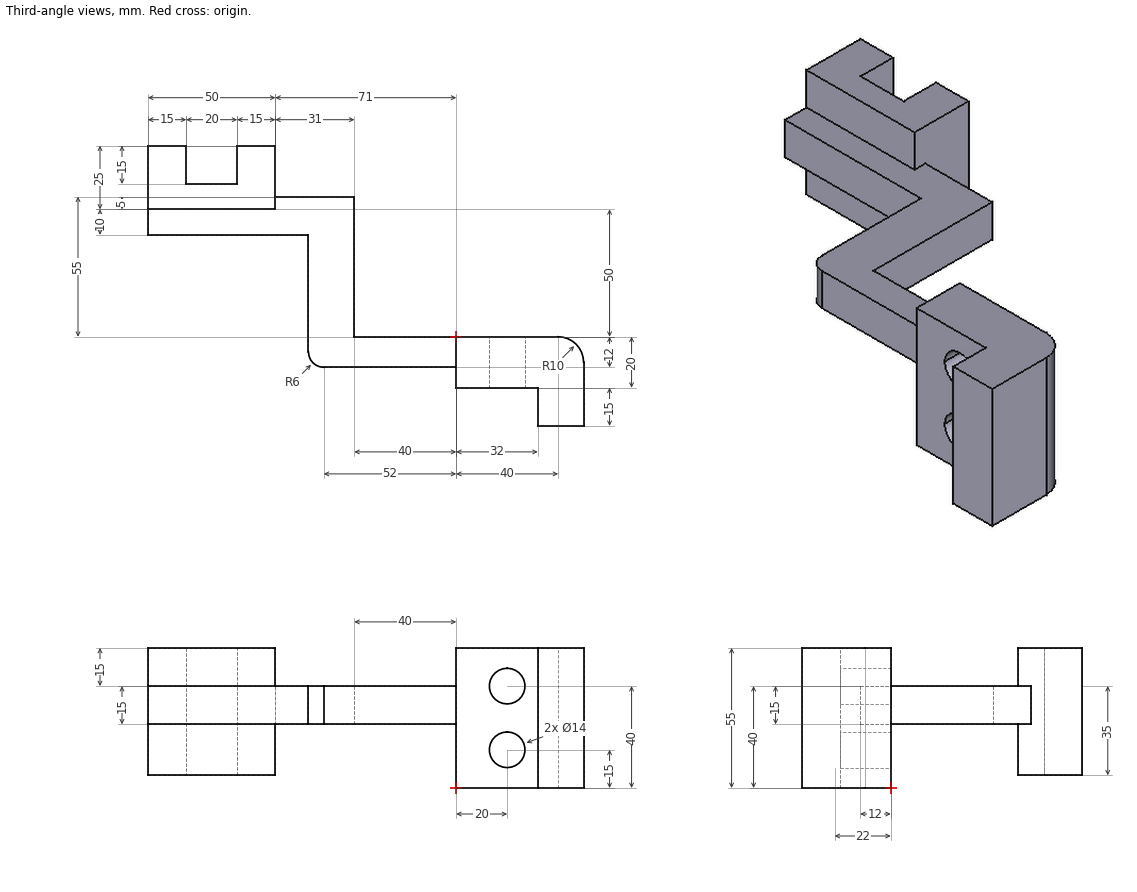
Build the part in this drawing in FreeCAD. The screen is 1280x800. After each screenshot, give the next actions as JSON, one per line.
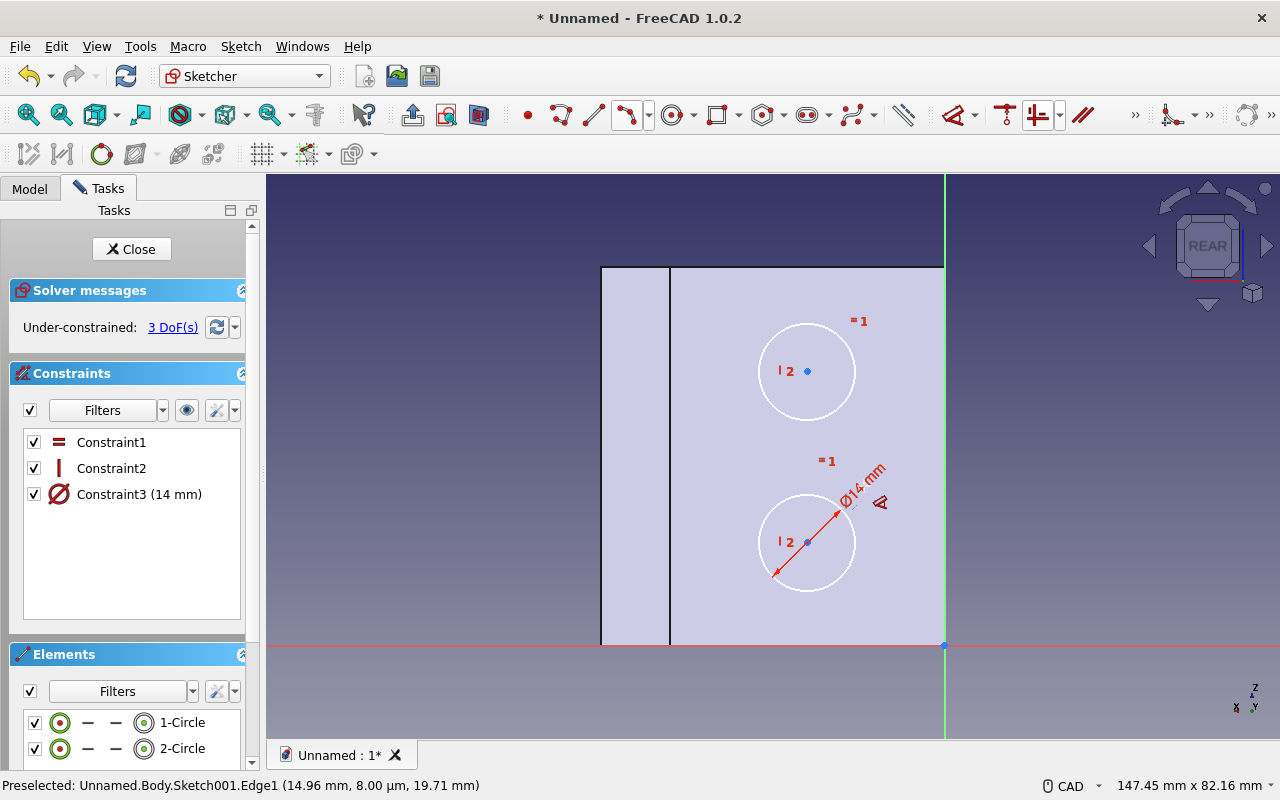
{"action": "left_click", "coordinate": [807, 543]}
{"action": "left_click", "coordinate": [876, 680]}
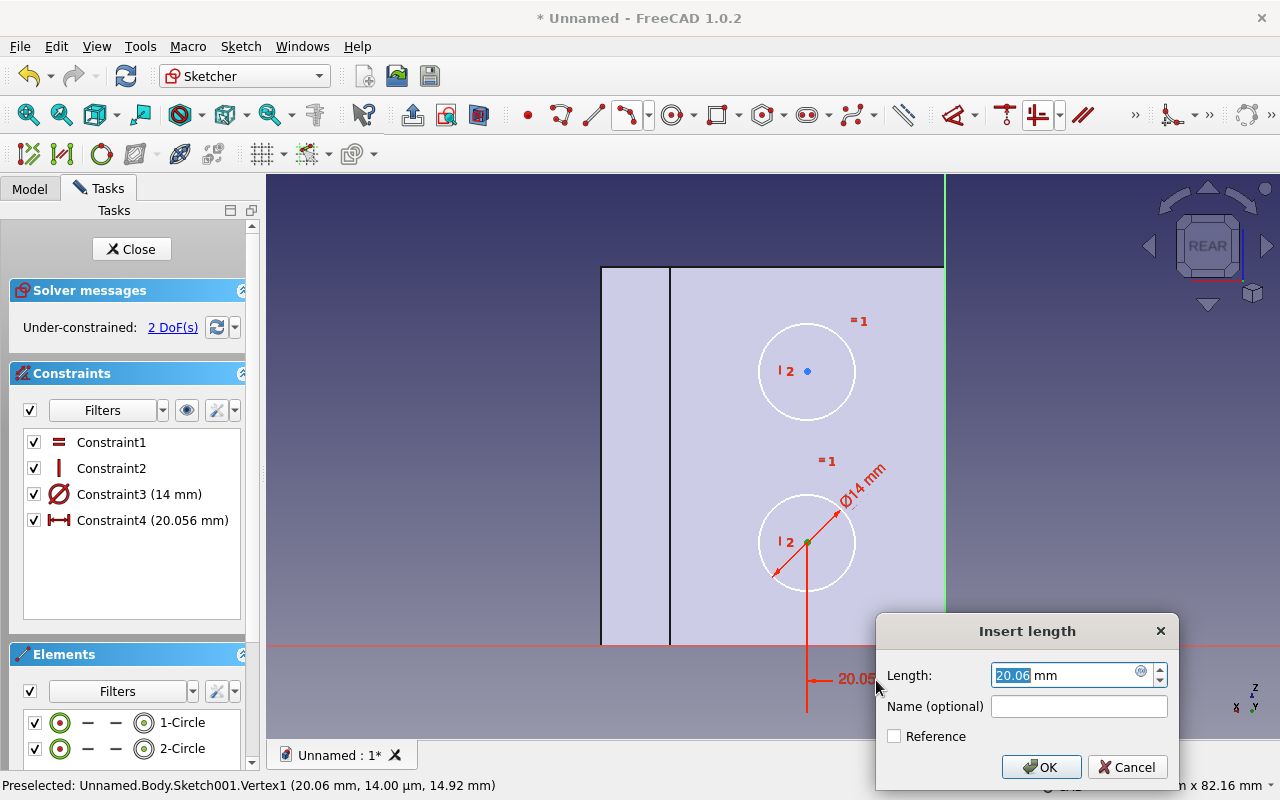
{"action": "type", "text": "20"}
{"action": "key", "text": "Return"}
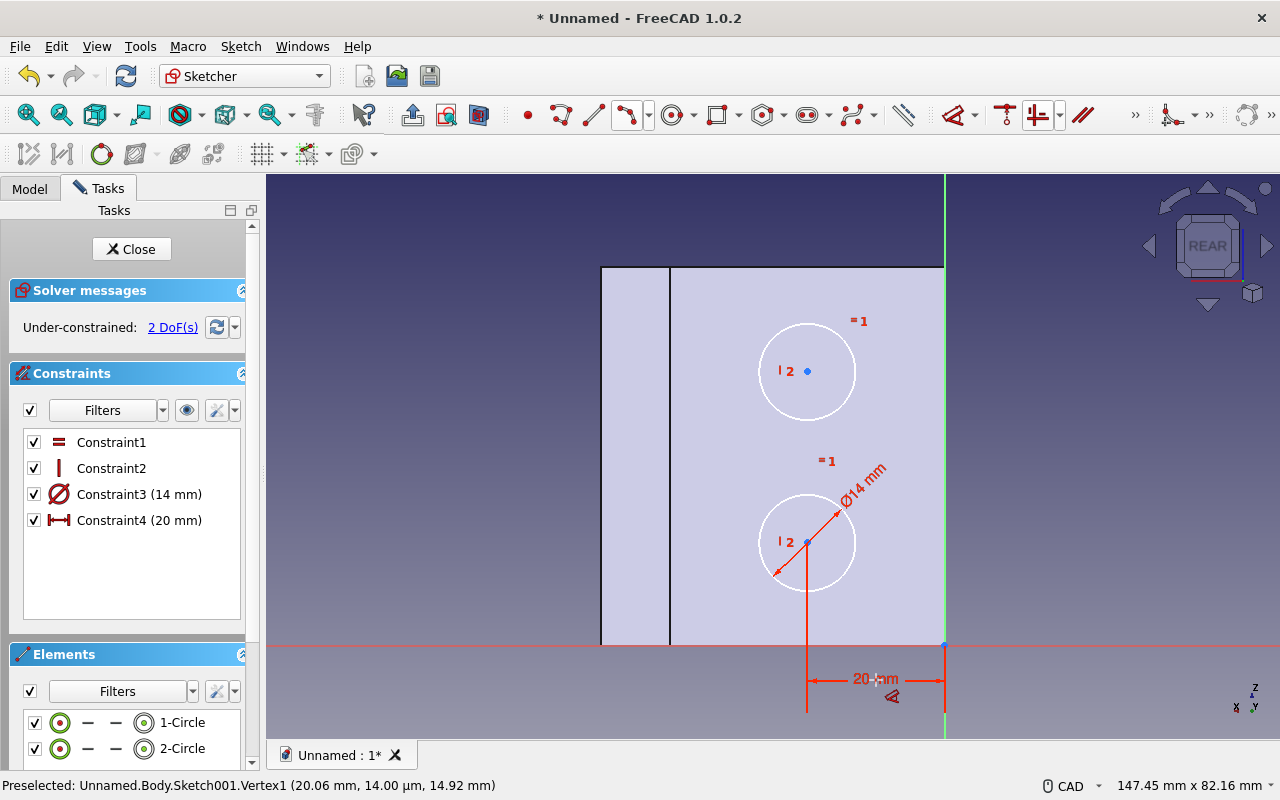
{"action": "left_click", "coordinate": [807, 543]}
{"action": "left_click", "coordinate": [979, 594]}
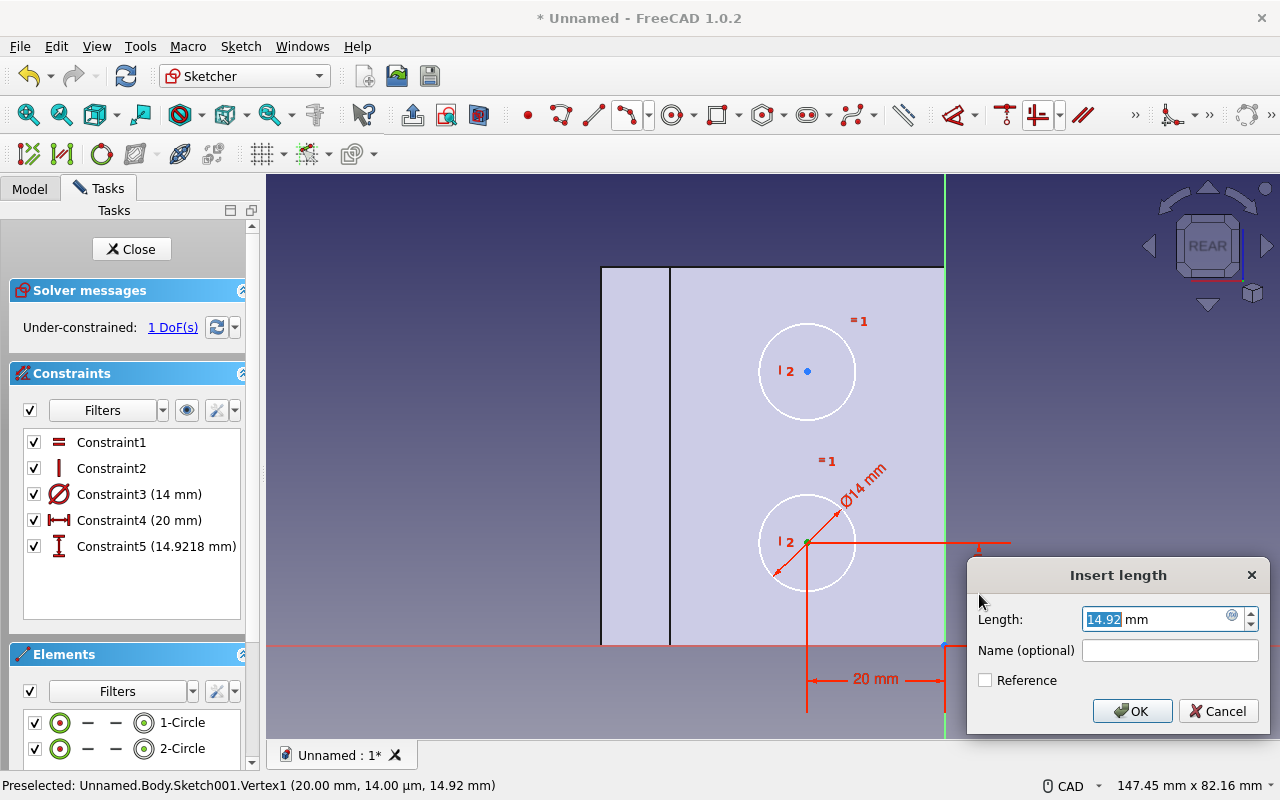
{"action": "type", "text": "15"}
{"action": "key", "text": "Return"}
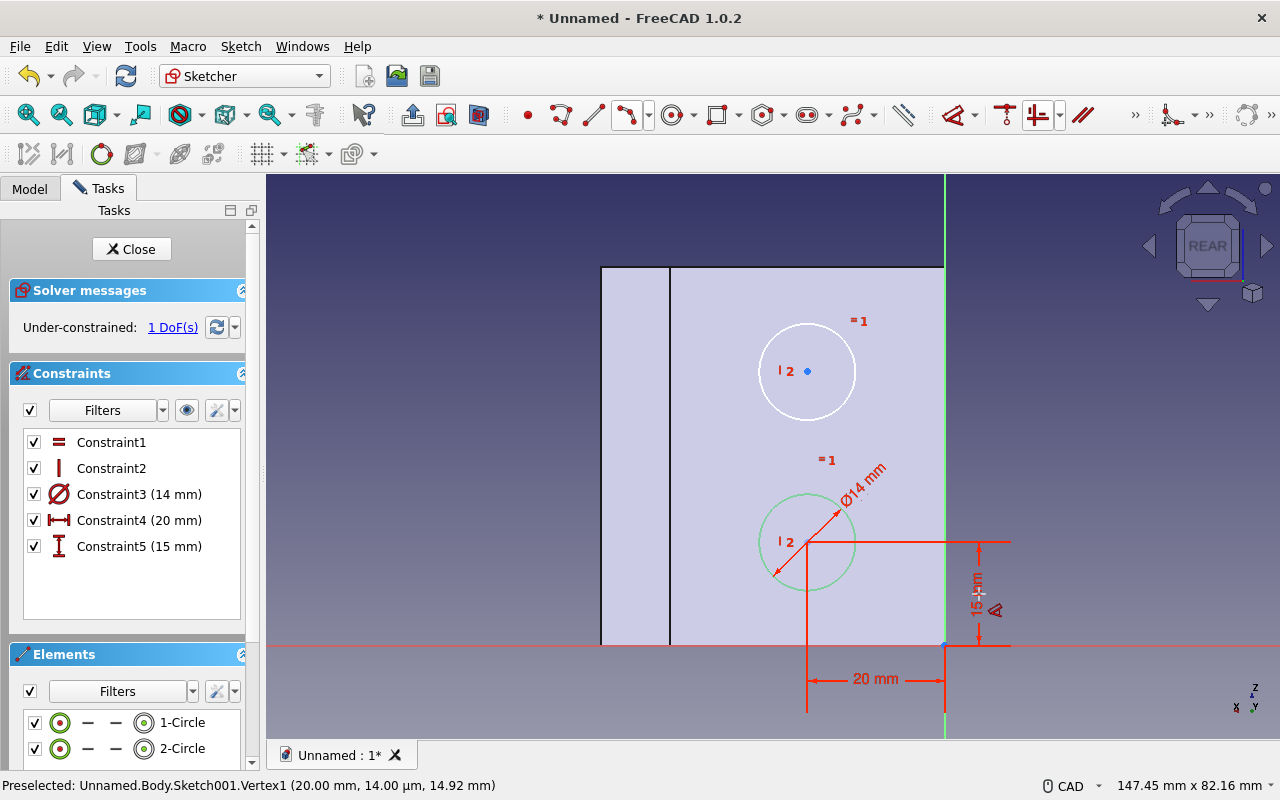
{"action": "left_click", "coordinate": [807, 372]}
{"action": "left_click", "coordinate": [979, 509]}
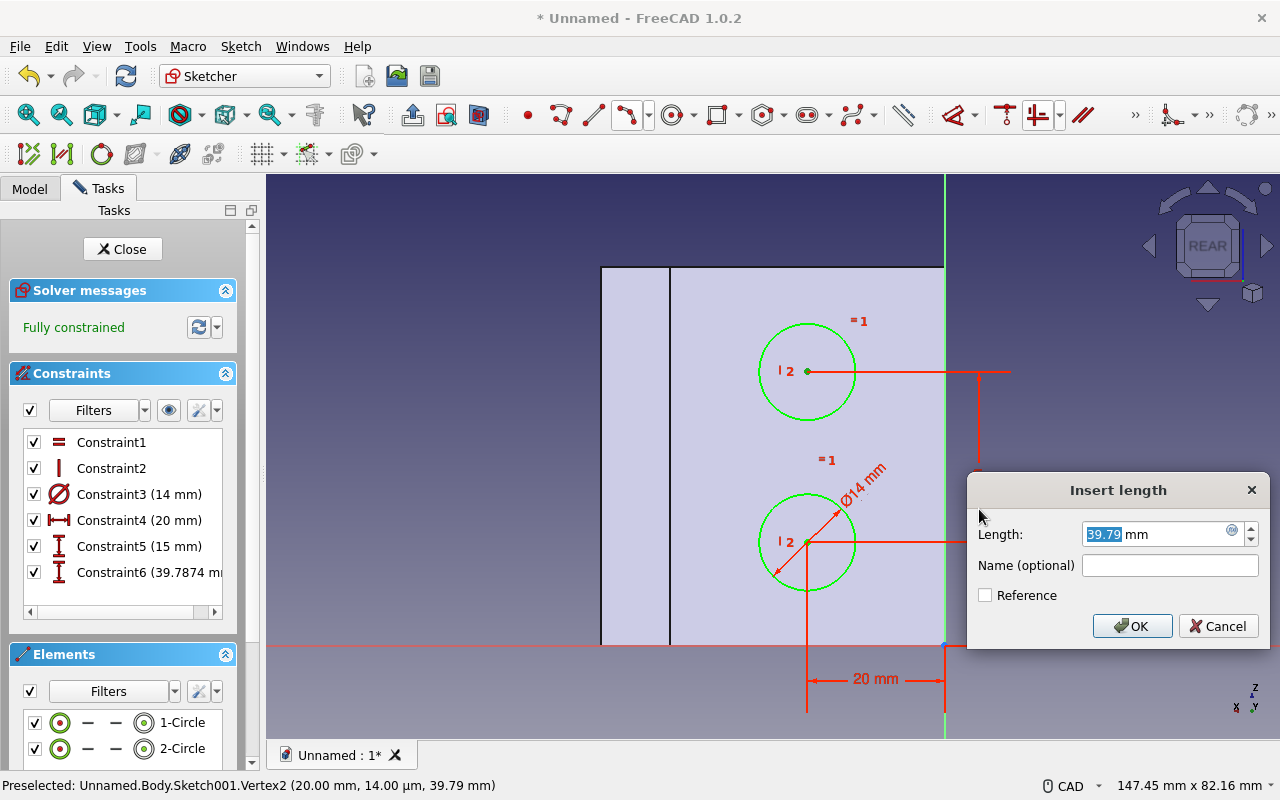
{"action": "type", "text": "40"}
{"action": "key", "text": "Return"}
{"action": "key", "text": "Escape"}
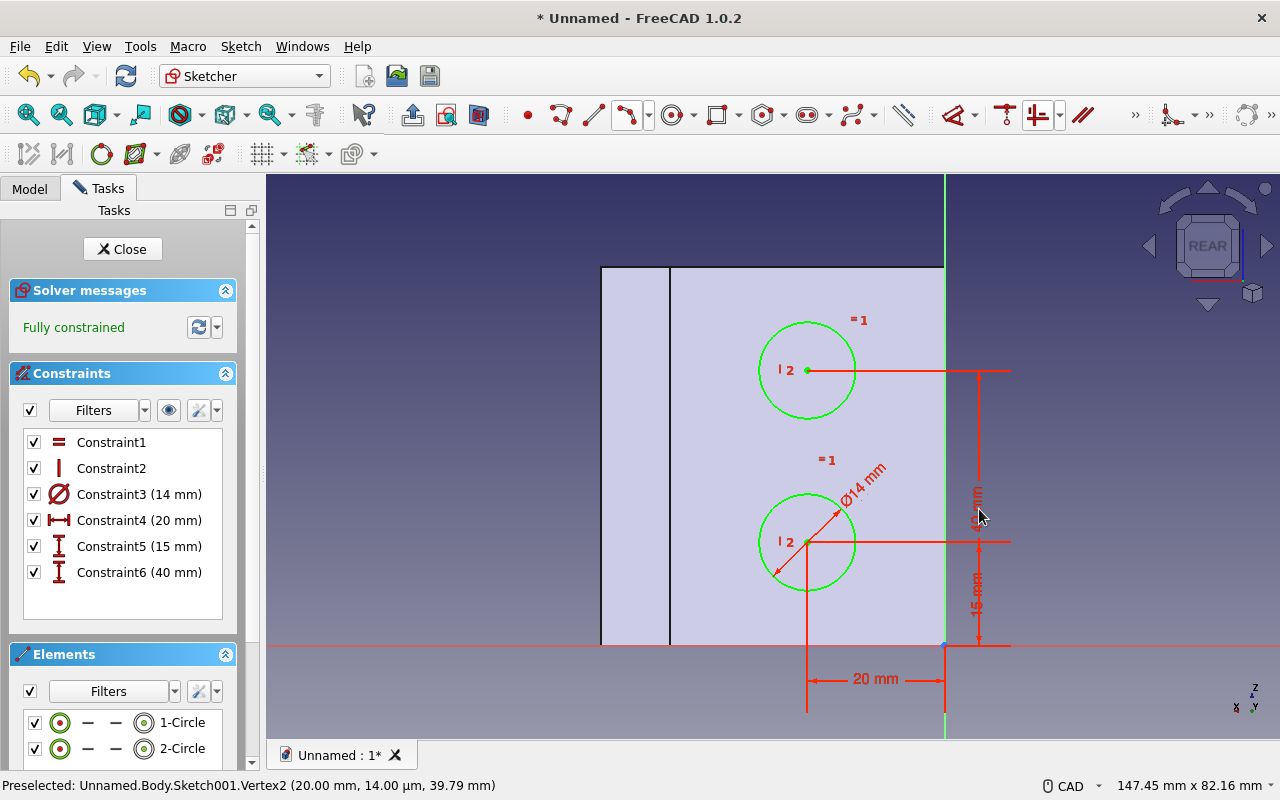
{"action": "left_click", "coordinate": [123, 249]}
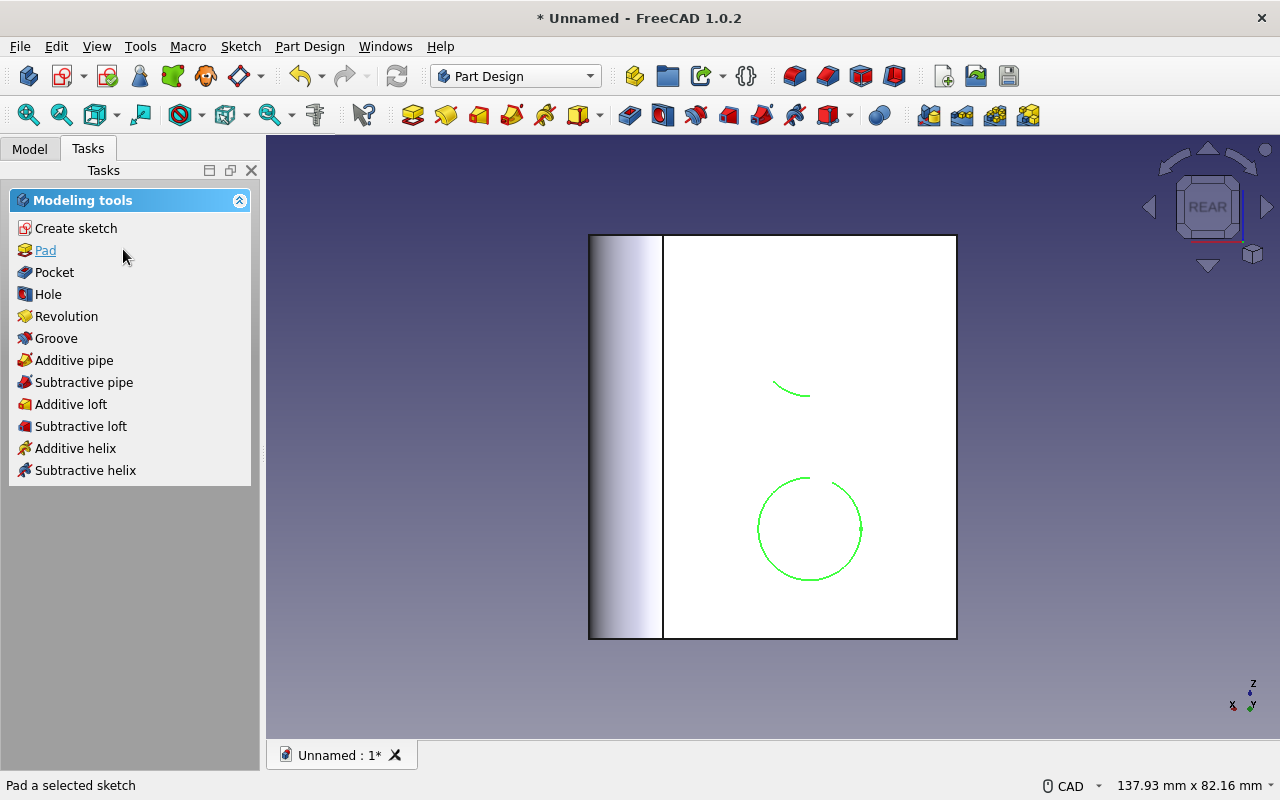
{"action": "left_click", "coordinate": [630, 116]}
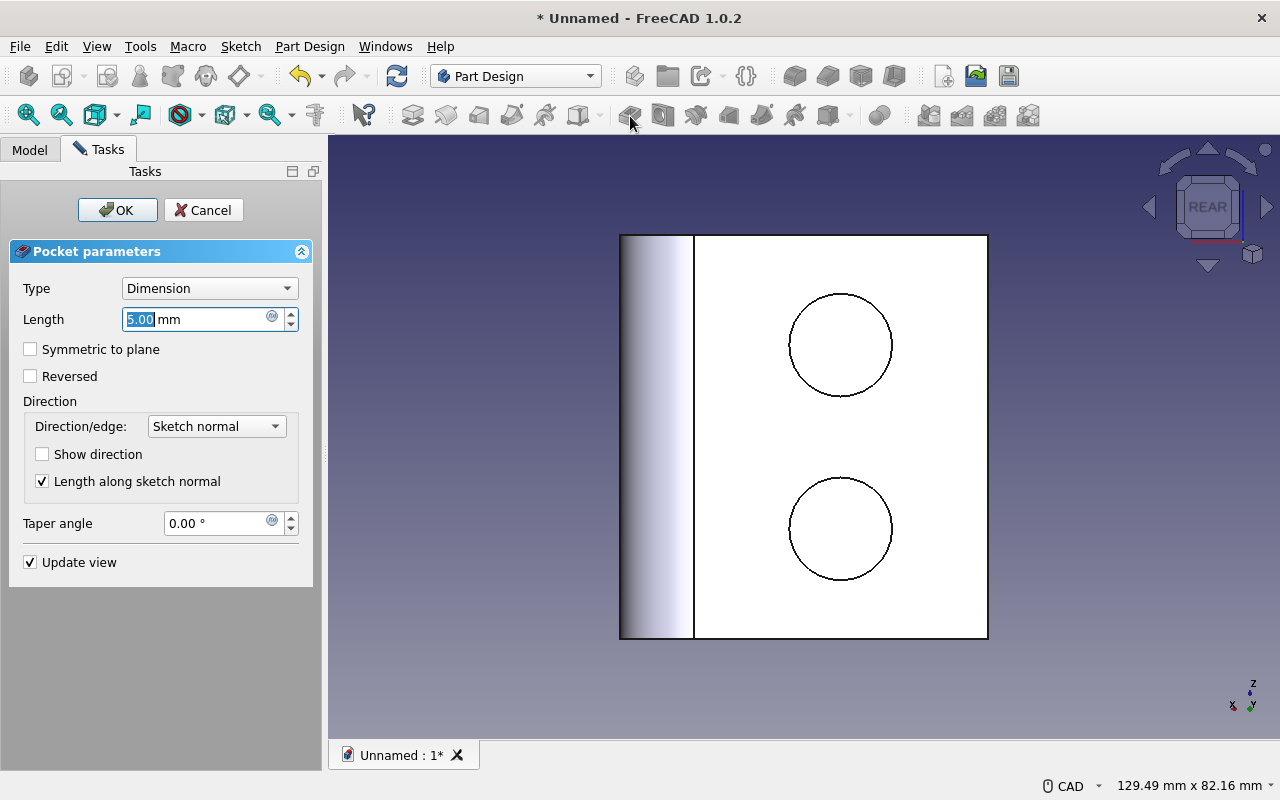
{"action": "type", "text": "22"}
{"action": "key", "text": "Tab"}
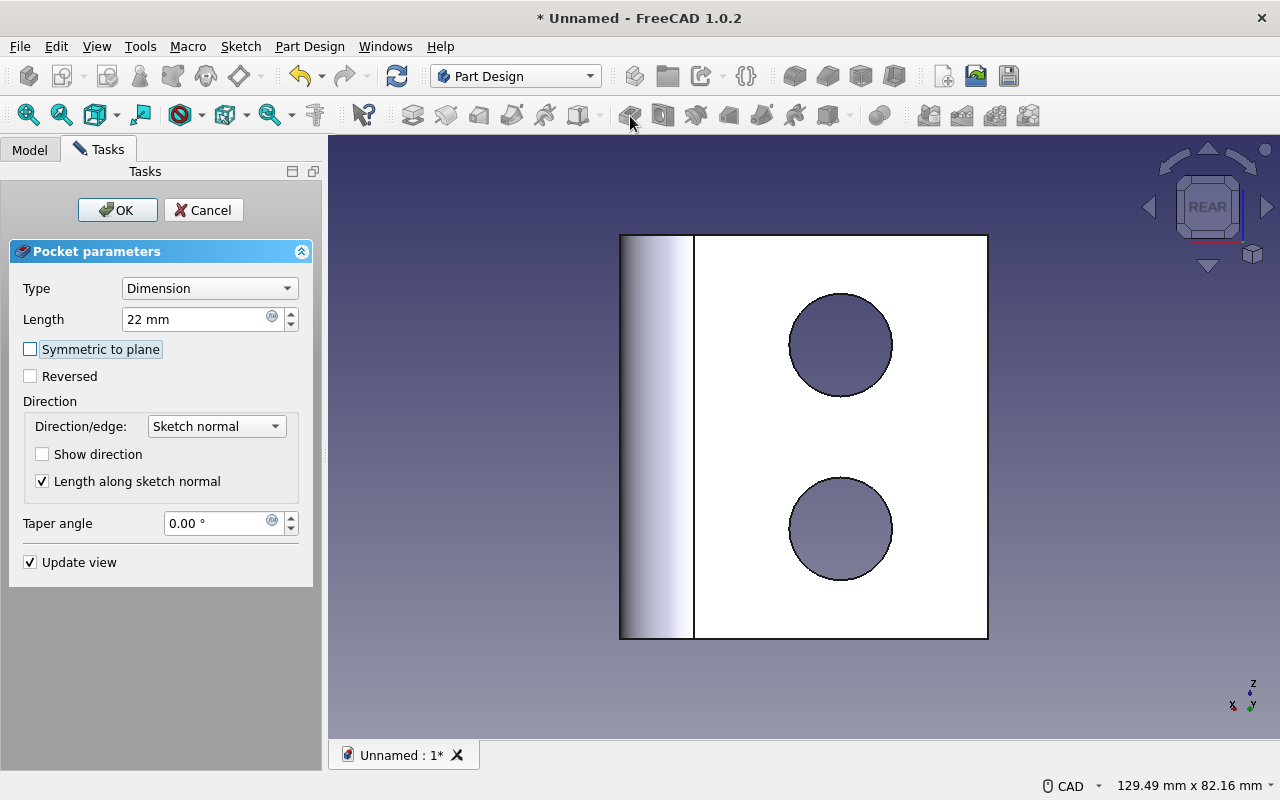
{"action": "left_click", "coordinate": [118, 210]}